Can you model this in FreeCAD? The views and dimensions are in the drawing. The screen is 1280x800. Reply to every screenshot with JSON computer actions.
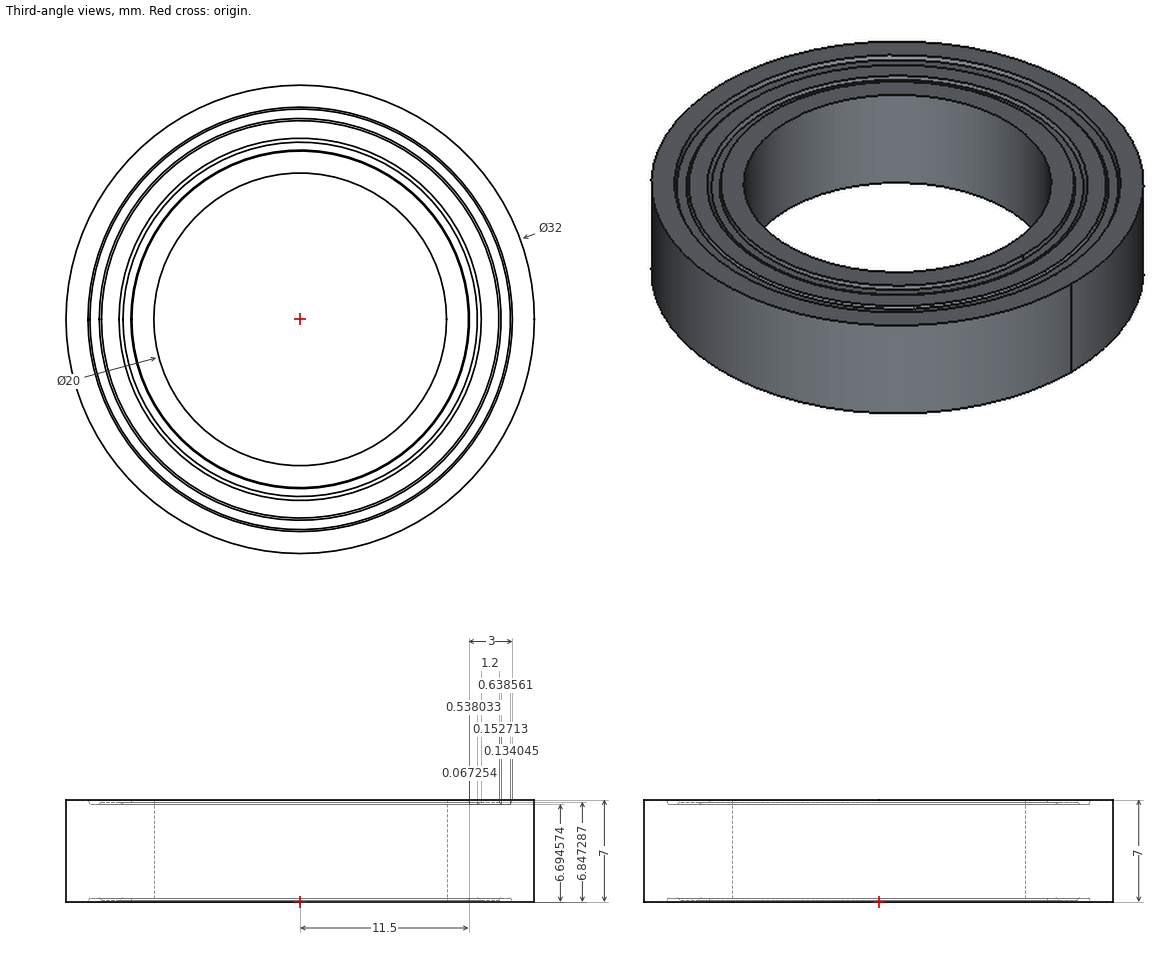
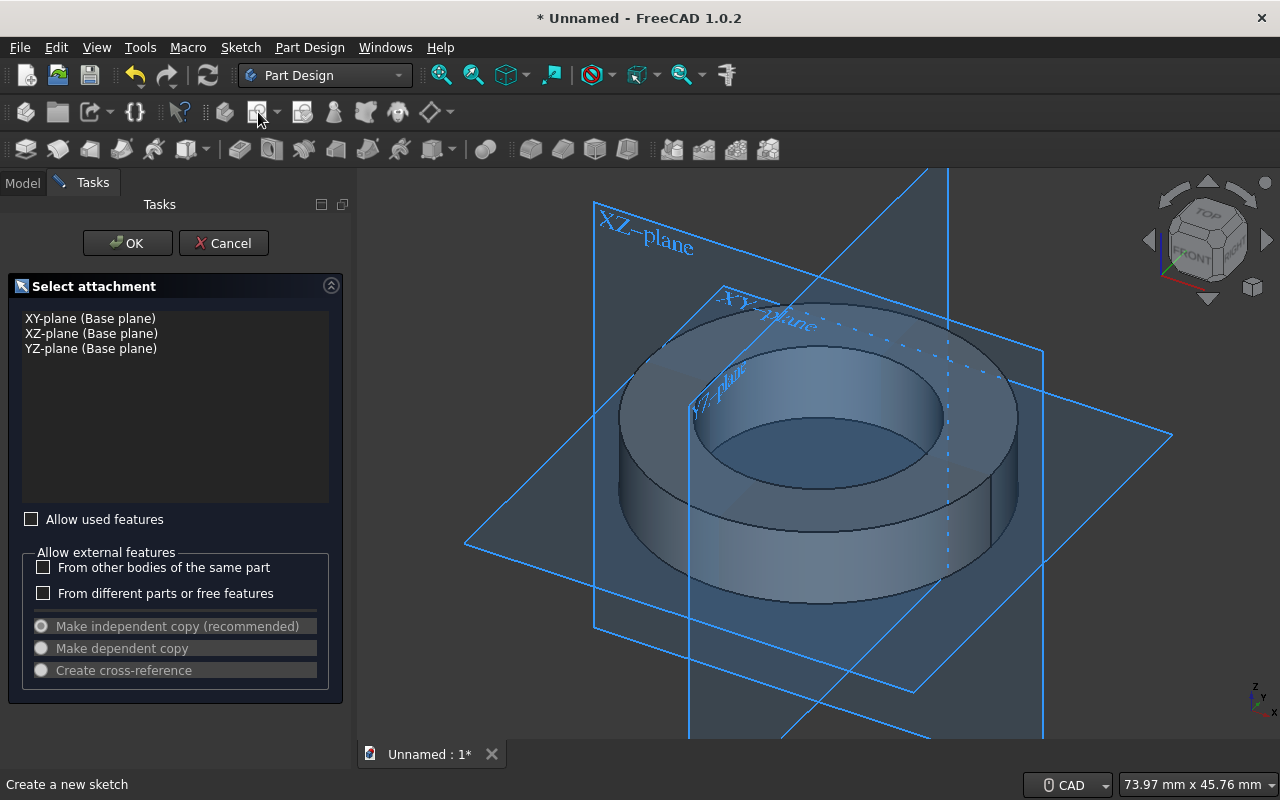
{"action": "left_click", "coordinate": [82, 334]}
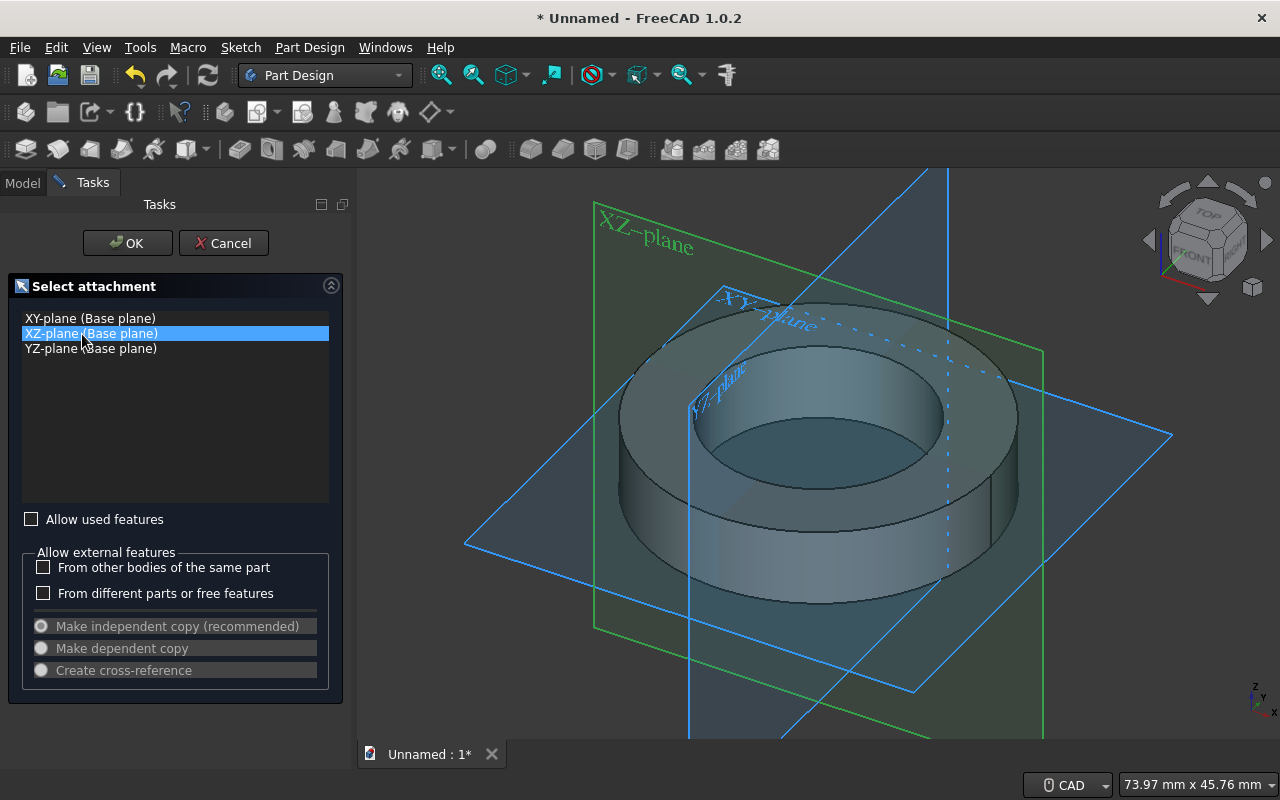
{"action": "left_click", "coordinate": [128, 243]}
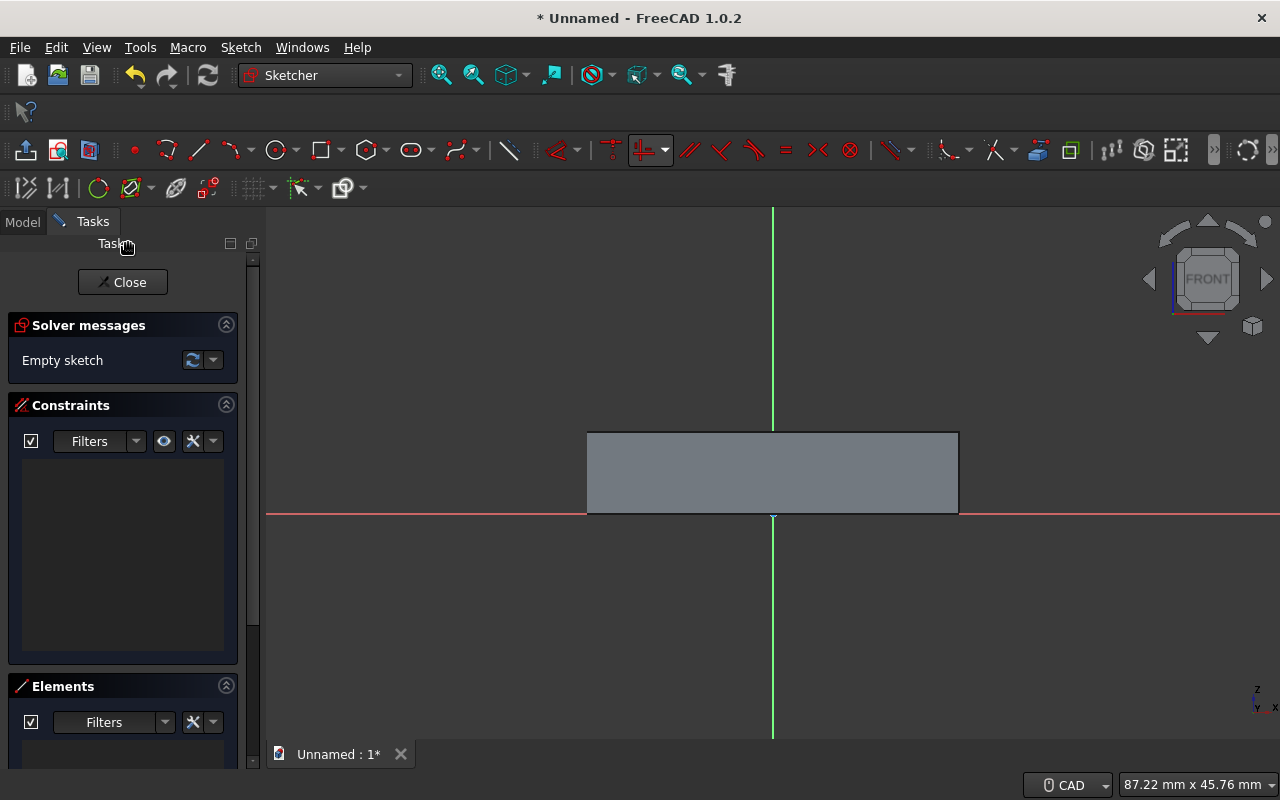
{"action": "key", "text": "q s"}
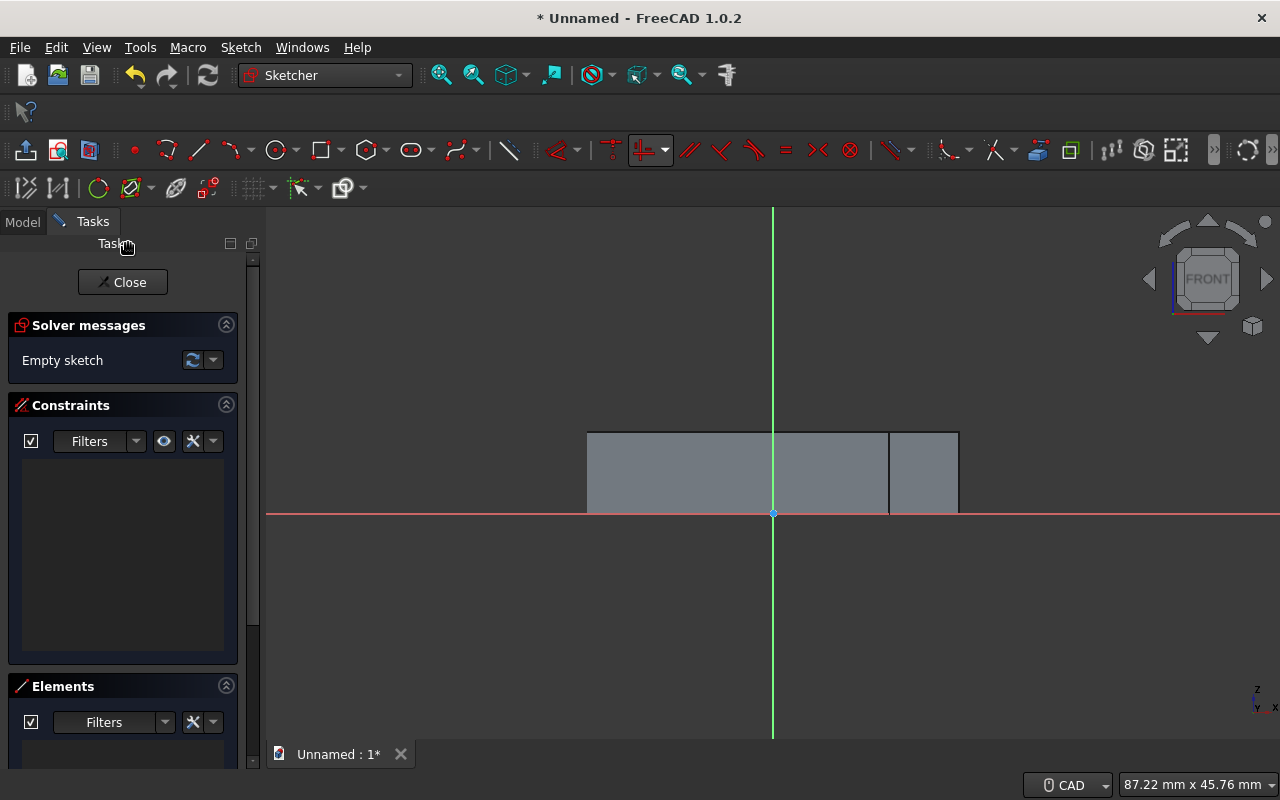
{"action": "scroll", "coordinate": [938, 432], "scroll_direction": "up", "scroll_amount": 14}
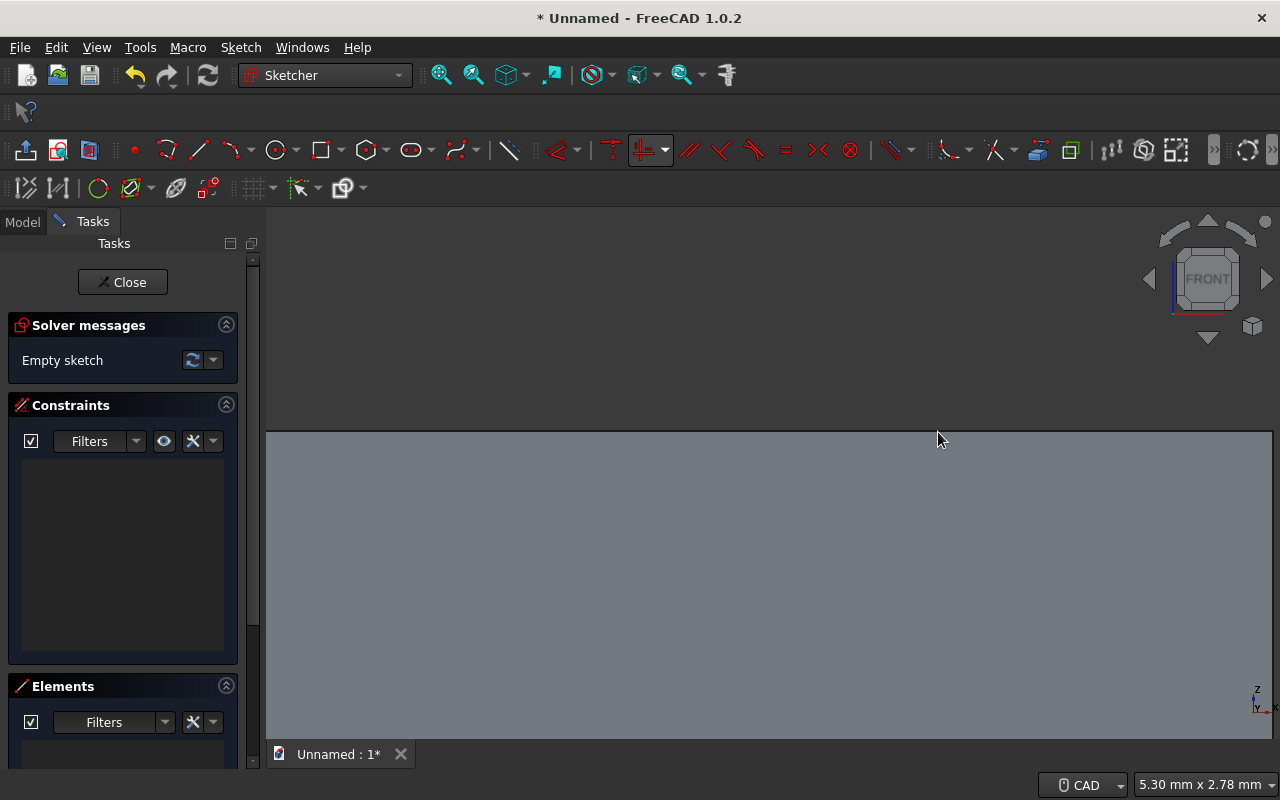
{"action": "key", "text": "g m"}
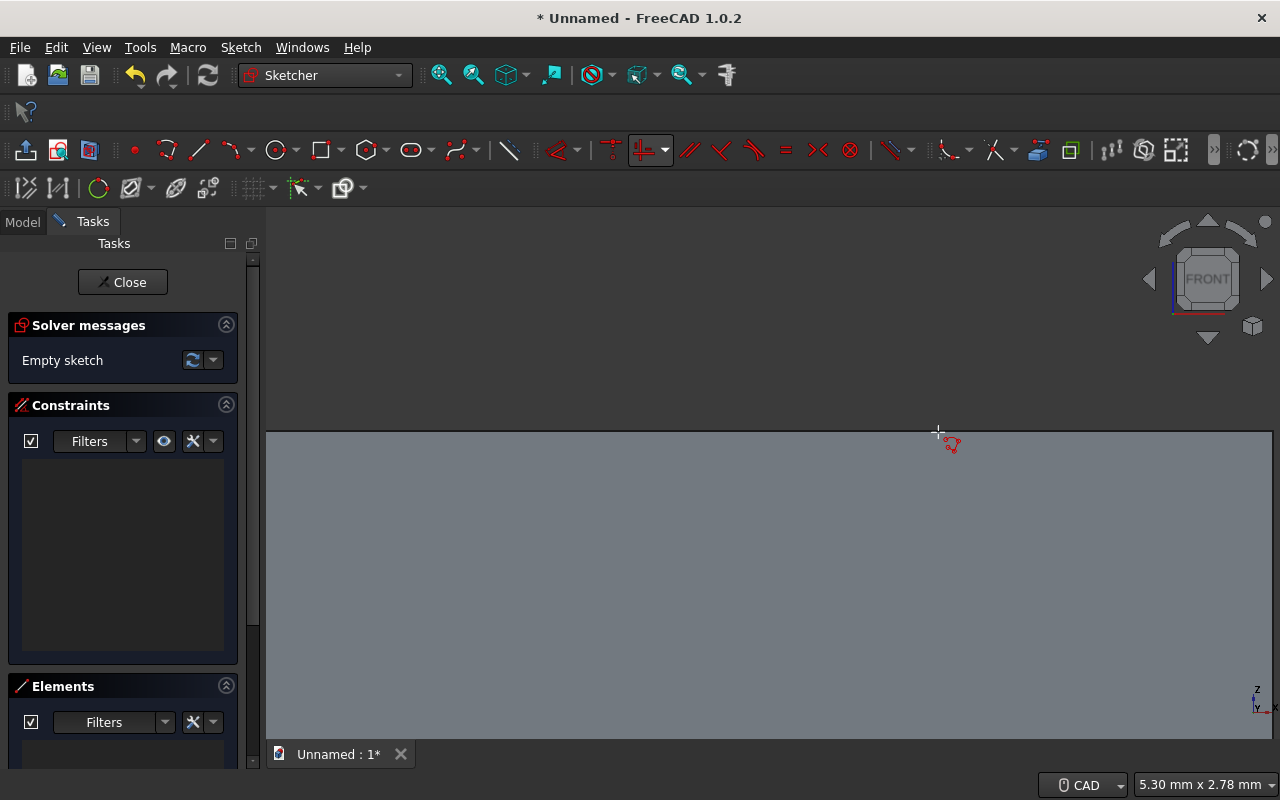
{"action": "left_click", "coordinate": [426, 489]}
{"action": "left_click", "coordinate": [413, 431]}
{"action": "left_click", "coordinate": [987, 431]}
{"action": "left_click", "coordinate": [961, 489]}
{"action": "left_click", "coordinate": [839, 489]}
{"action": "left_click", "coordinate": [810, 460]}
{"action": "left_click", "coordinate": [580, 460]}
{"action": "left_click", "coordinate": [529, 489]}
{"action": "left_click", "coordinate": [426, 490]}
{"action": "key", "text": "Escape"}
{"action": "key", "text": "Escape"}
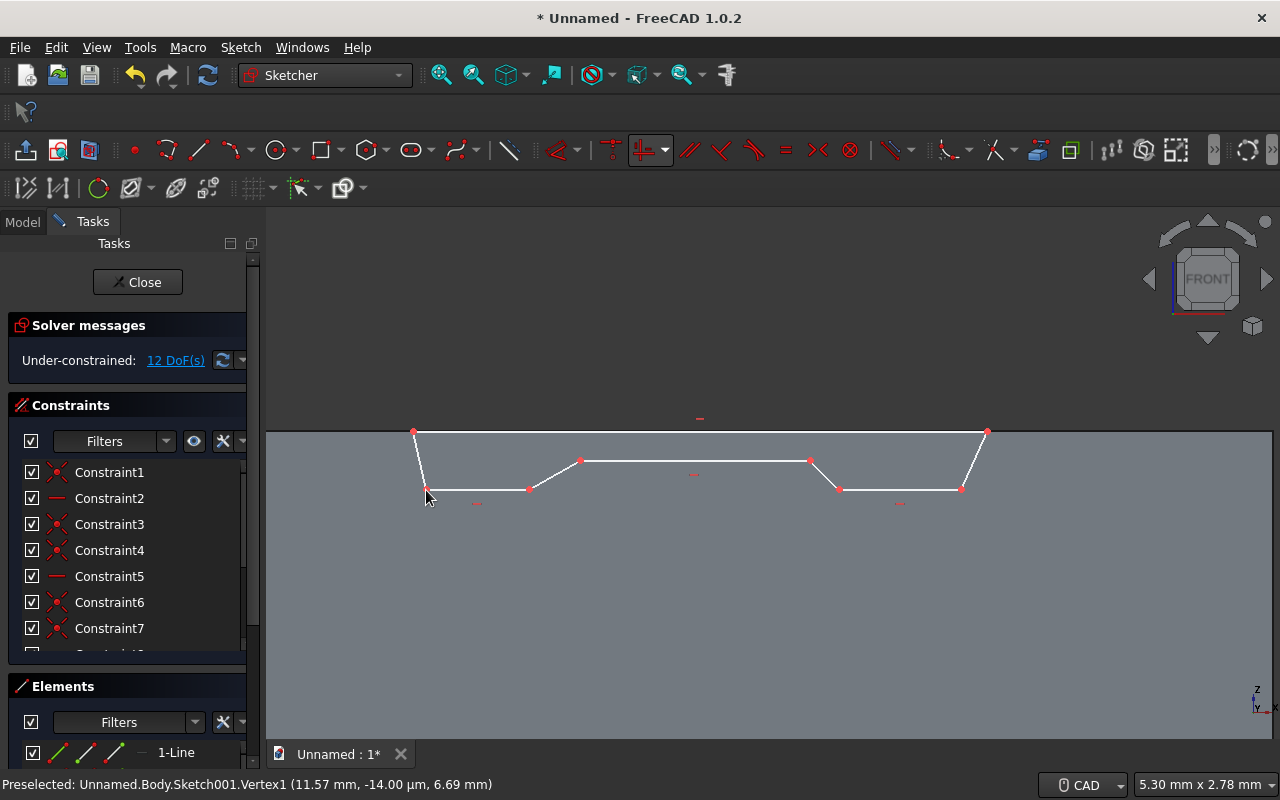
{"action": "key", "text": "d"}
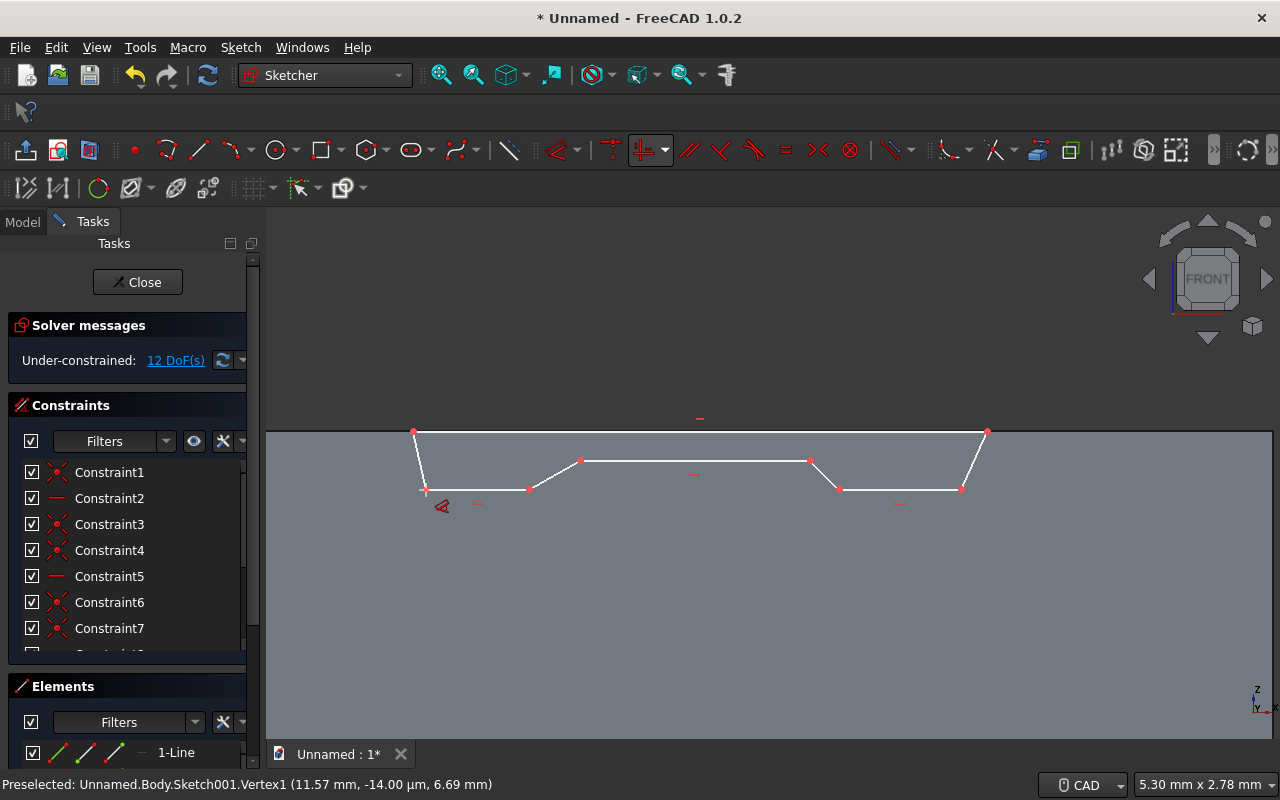
{"action": "left_click", "coordinate": [585, 432]}
{"action": "left_click", "coordinate": [700, 398]}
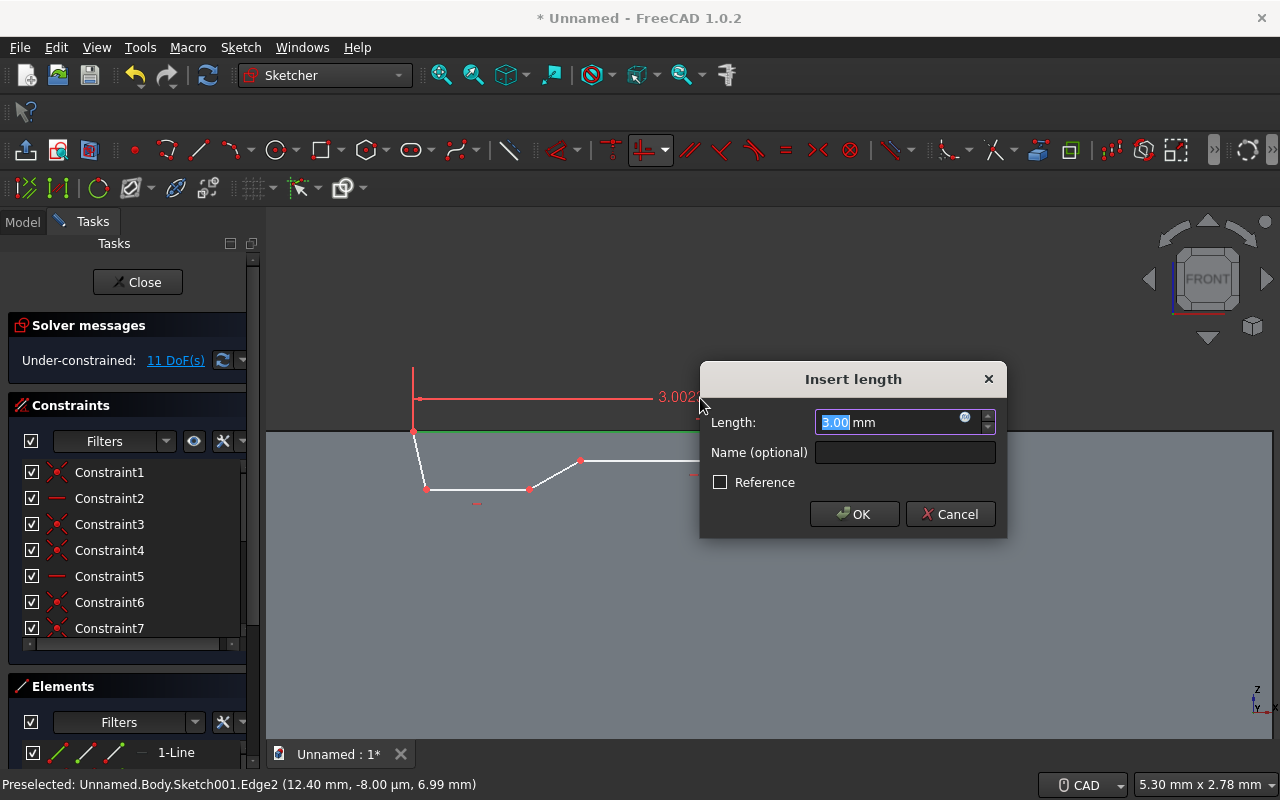
{"action": "type", "text": "3"}
{"action": "key", "text": "Return"}